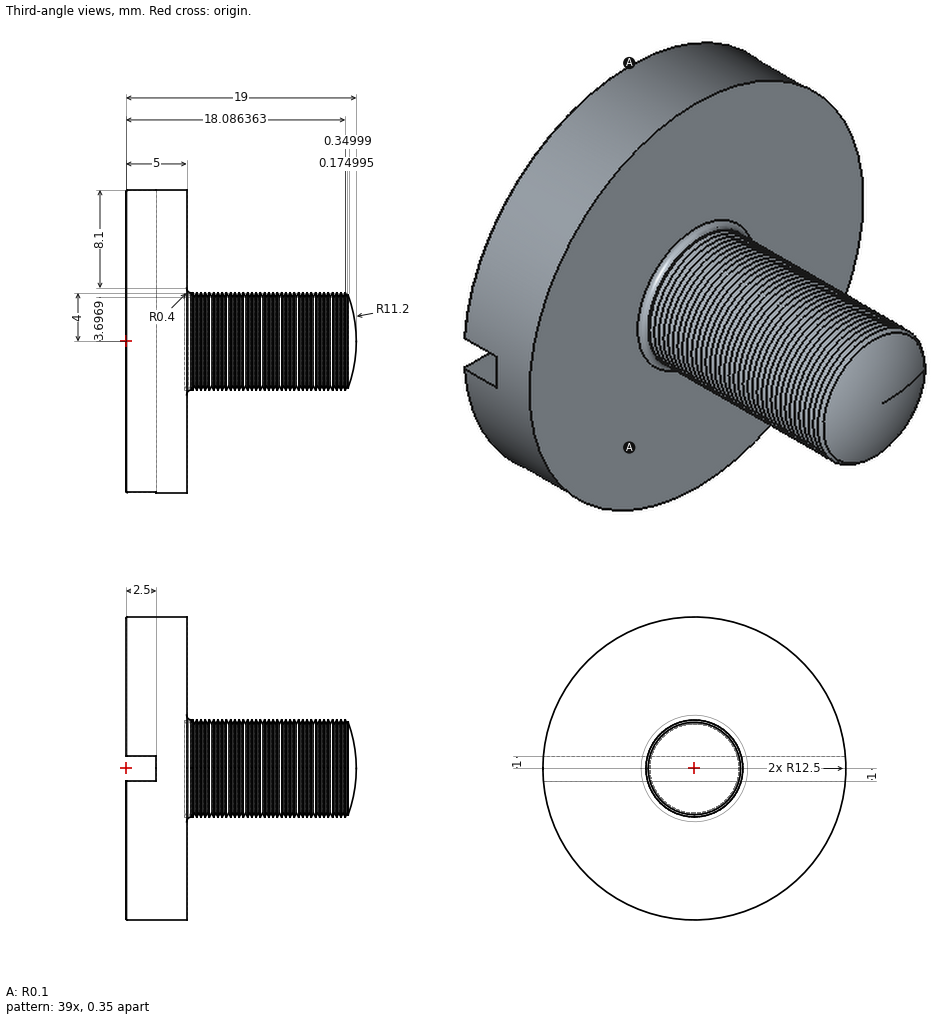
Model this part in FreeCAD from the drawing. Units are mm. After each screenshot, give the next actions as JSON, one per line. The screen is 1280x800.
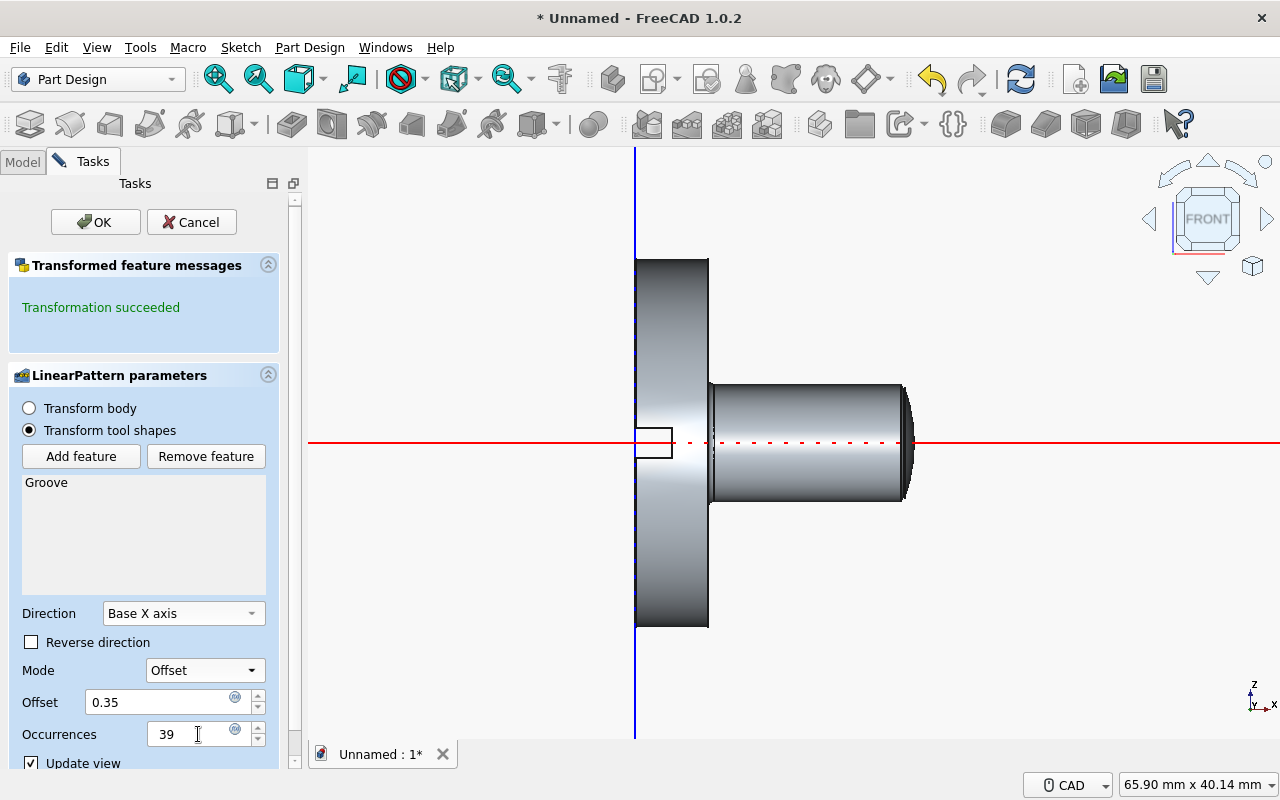
{"action": "left_click", "coordinate": [30, 642]}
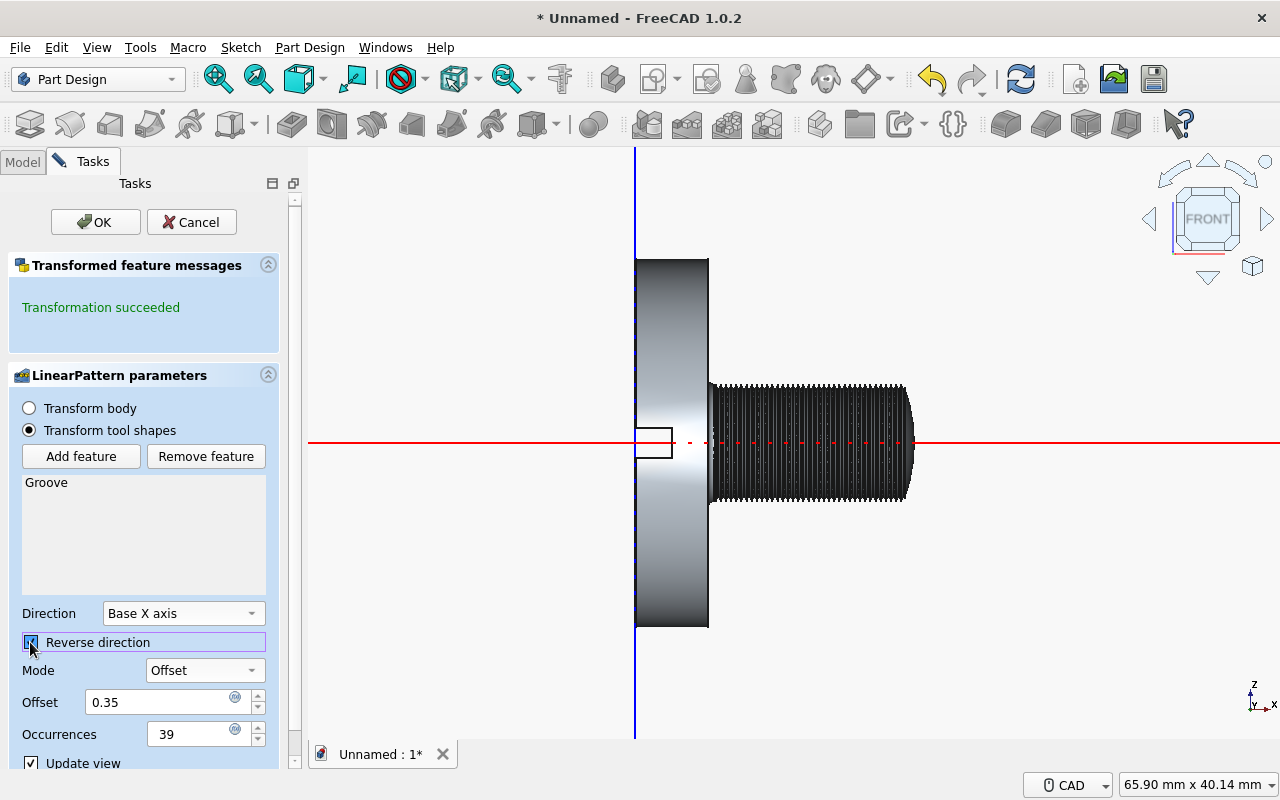
{"action": "left_click", "coordinate": [96, 222]}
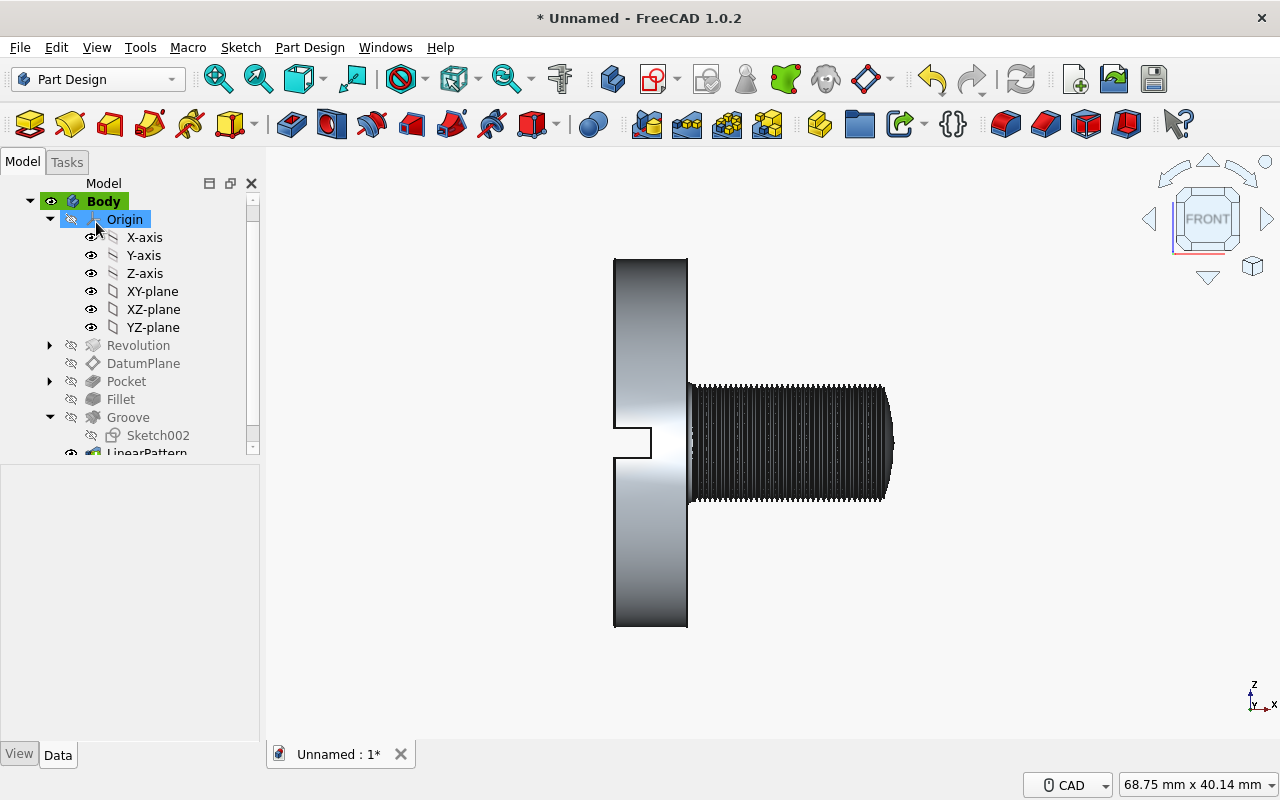
{"action": "key", "text": "0"}